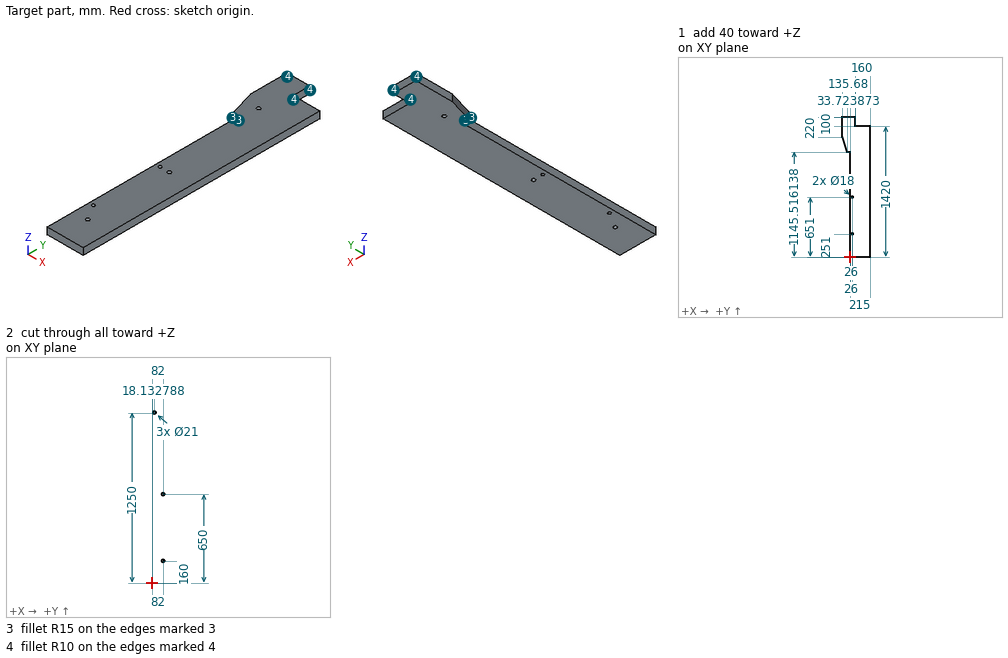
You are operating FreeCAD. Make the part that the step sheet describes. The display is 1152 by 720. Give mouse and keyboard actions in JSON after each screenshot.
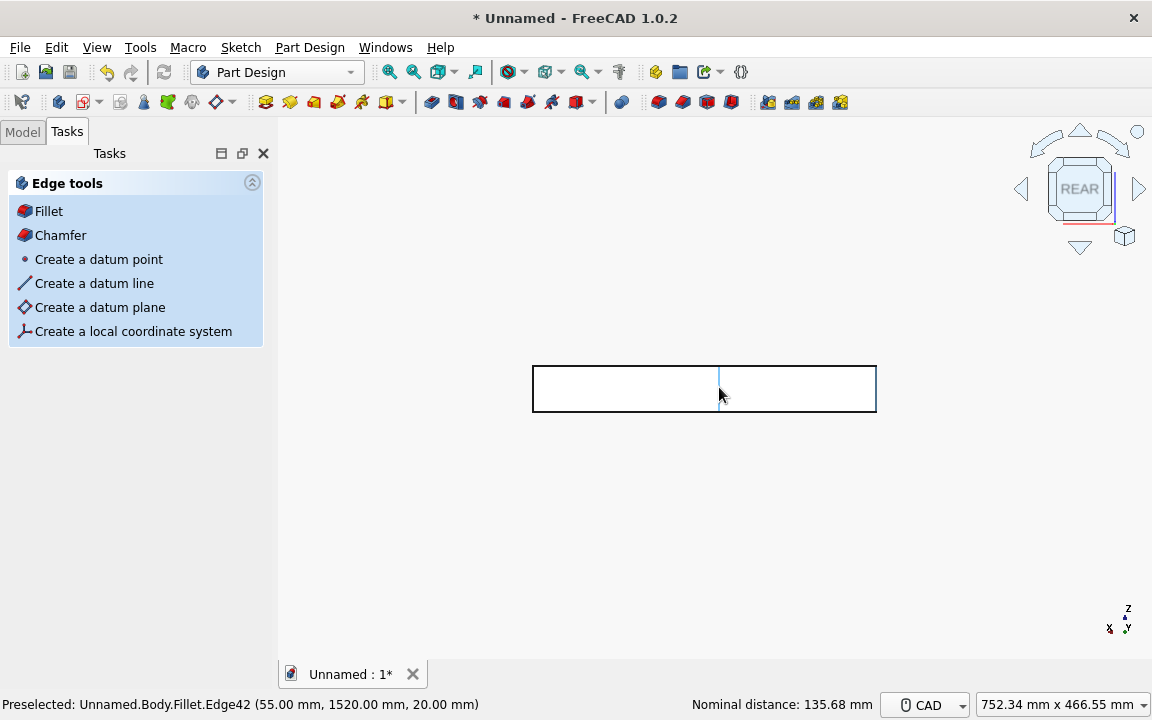
{"action": "key", "text": "v f"}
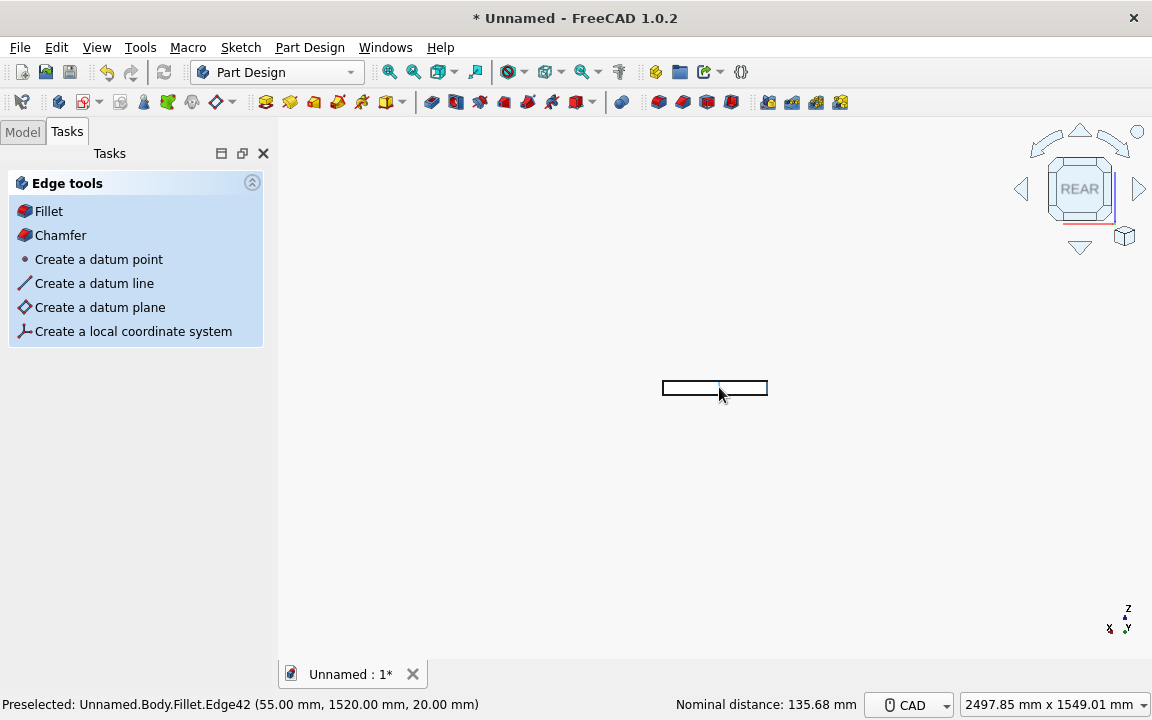
{"action": "key", "text": "6"}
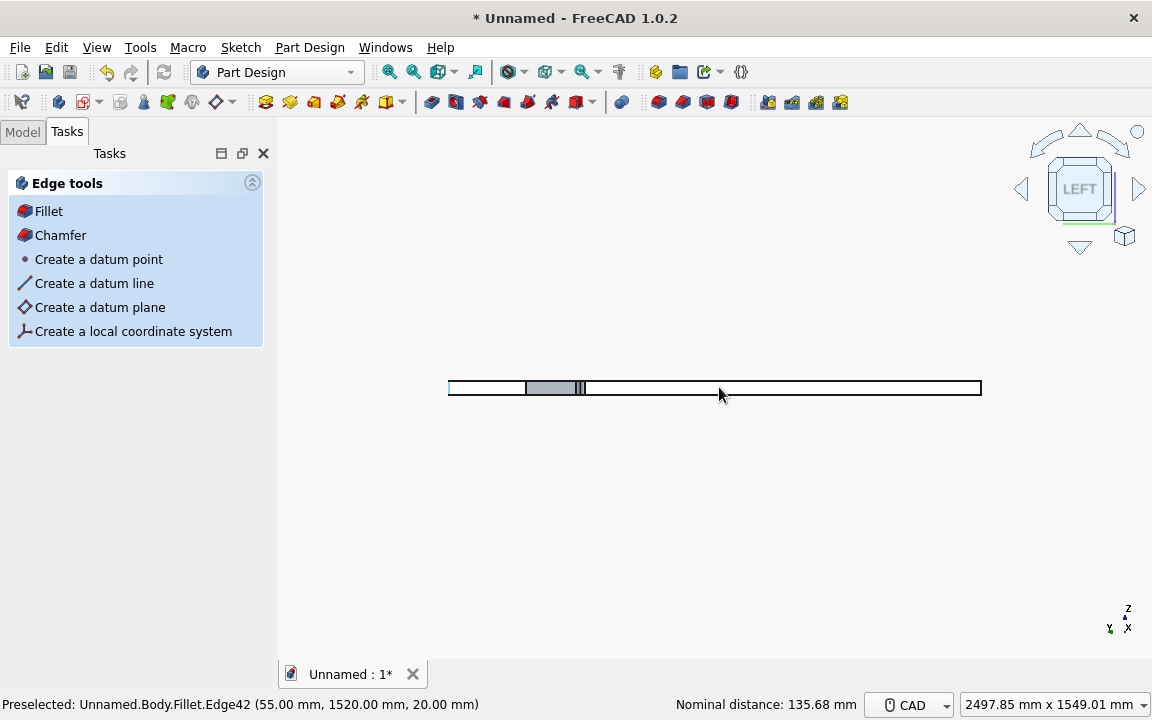
{"action": "scroll", "coordinate": [484, 387], "scroll_direction": "up", "scroll_amount": 6}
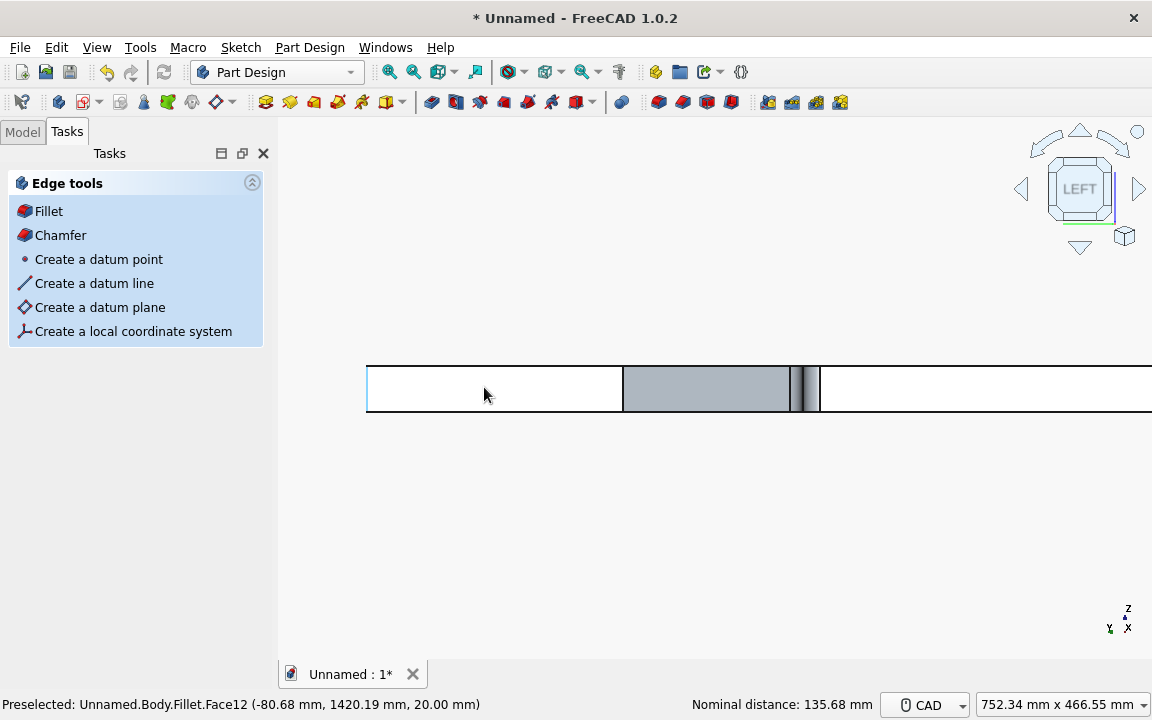
{"action": "key", "text": "v f"}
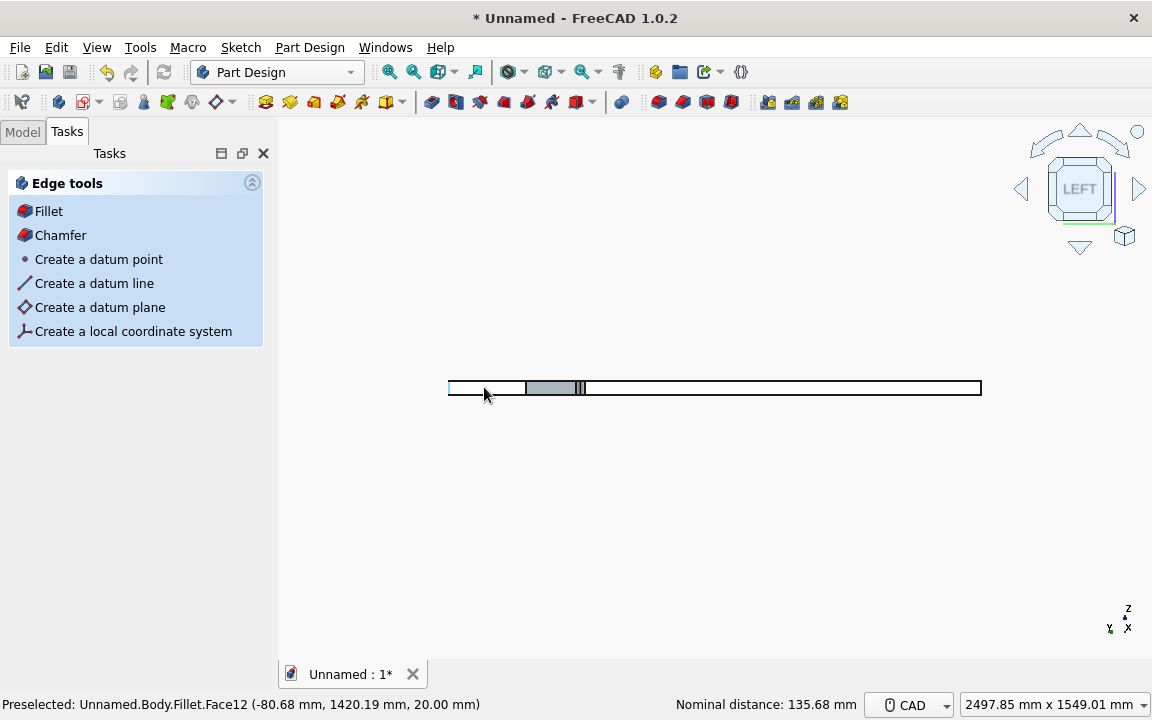
{"action": "key", "text": "v 3"}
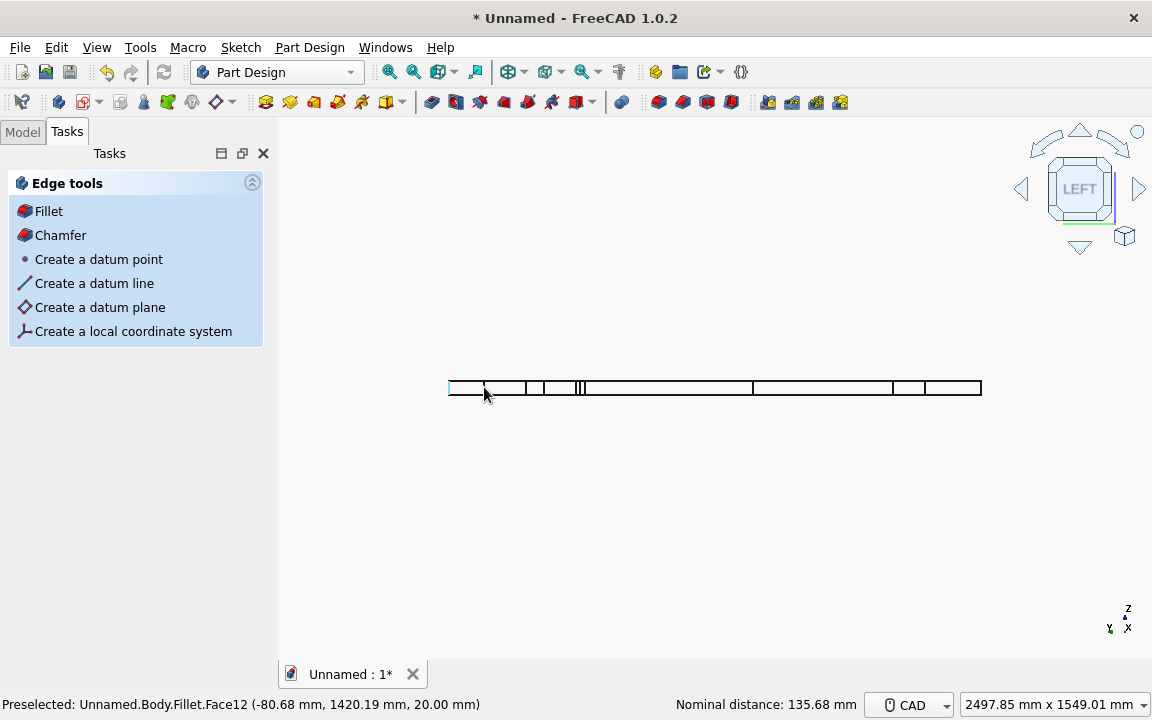
{"action": "key", "text": "0"}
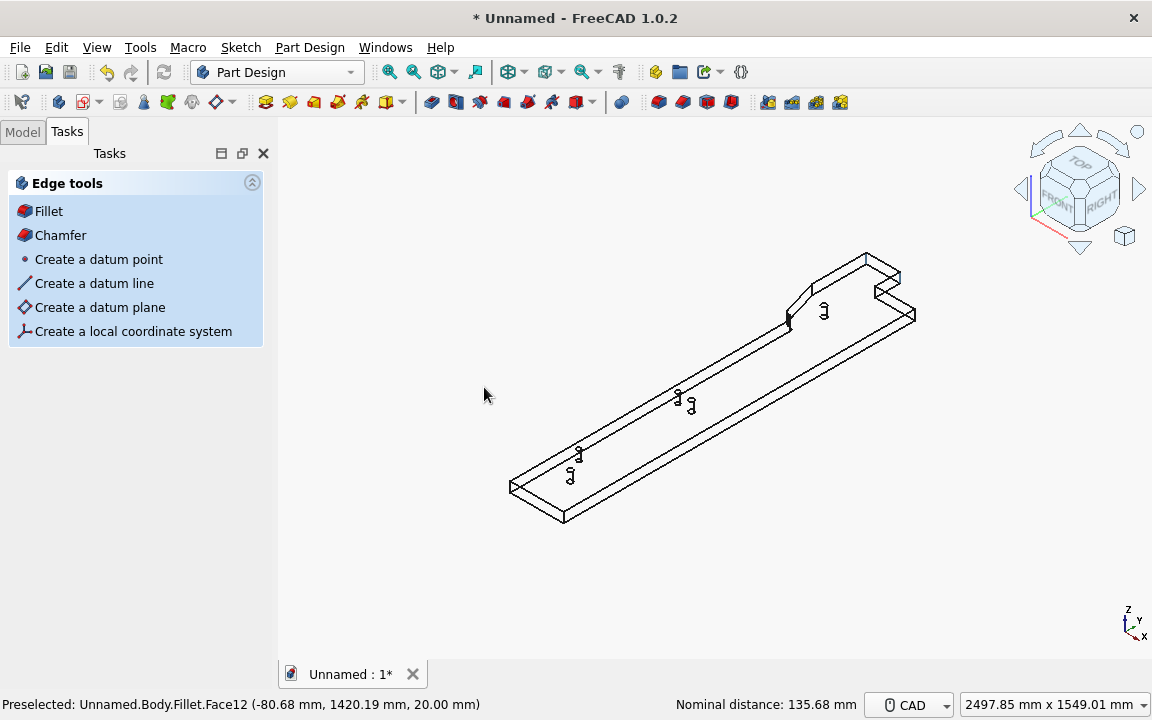
{"action": "left_click", "coordinate": [875, 293], "text": "ctrl"}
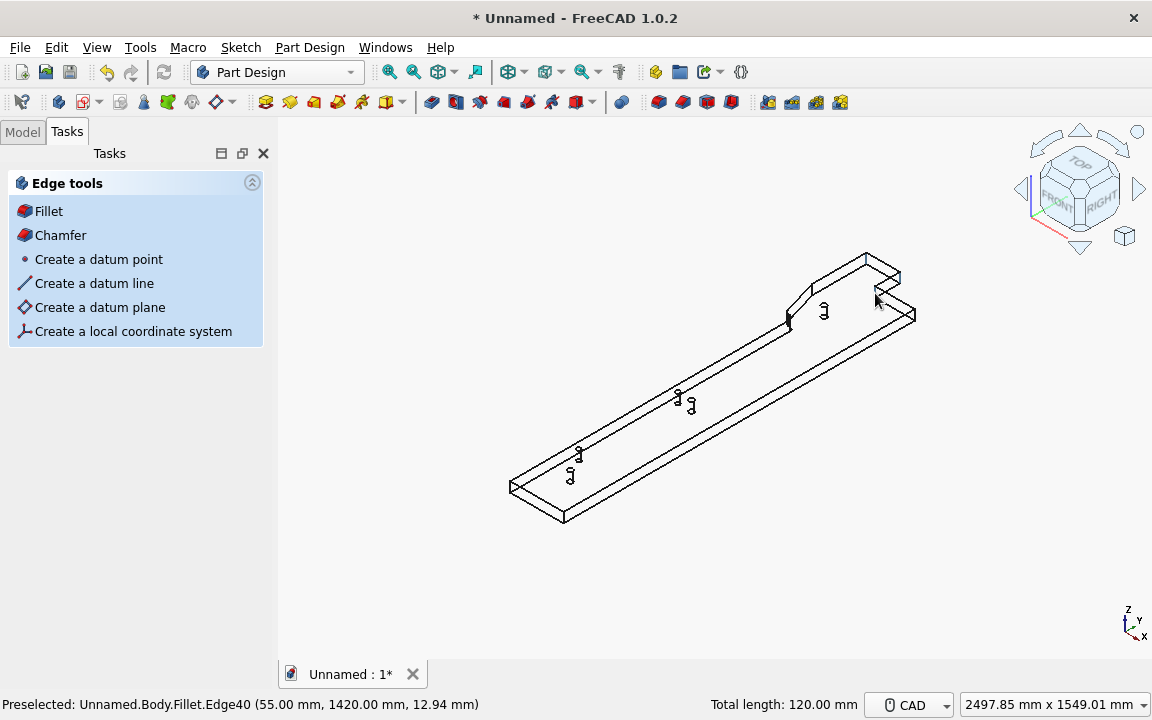
{"action": "key", "text": "v 1"}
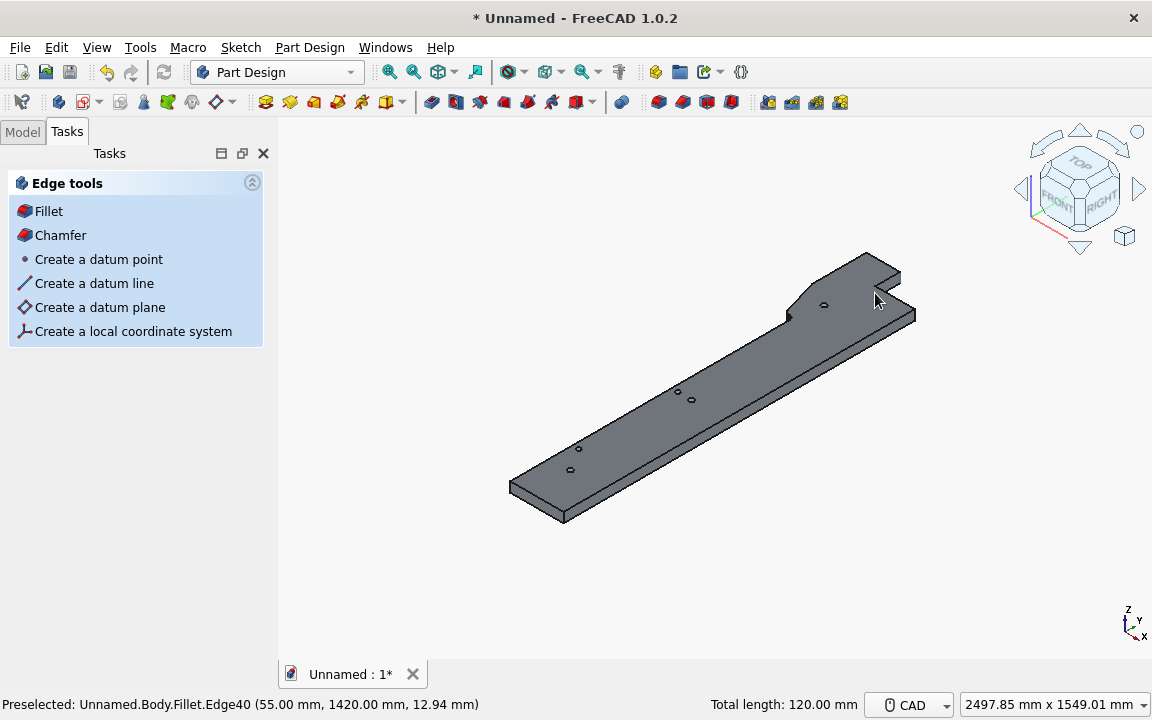
{"action": "left_click", "coordinate": [660, 102]}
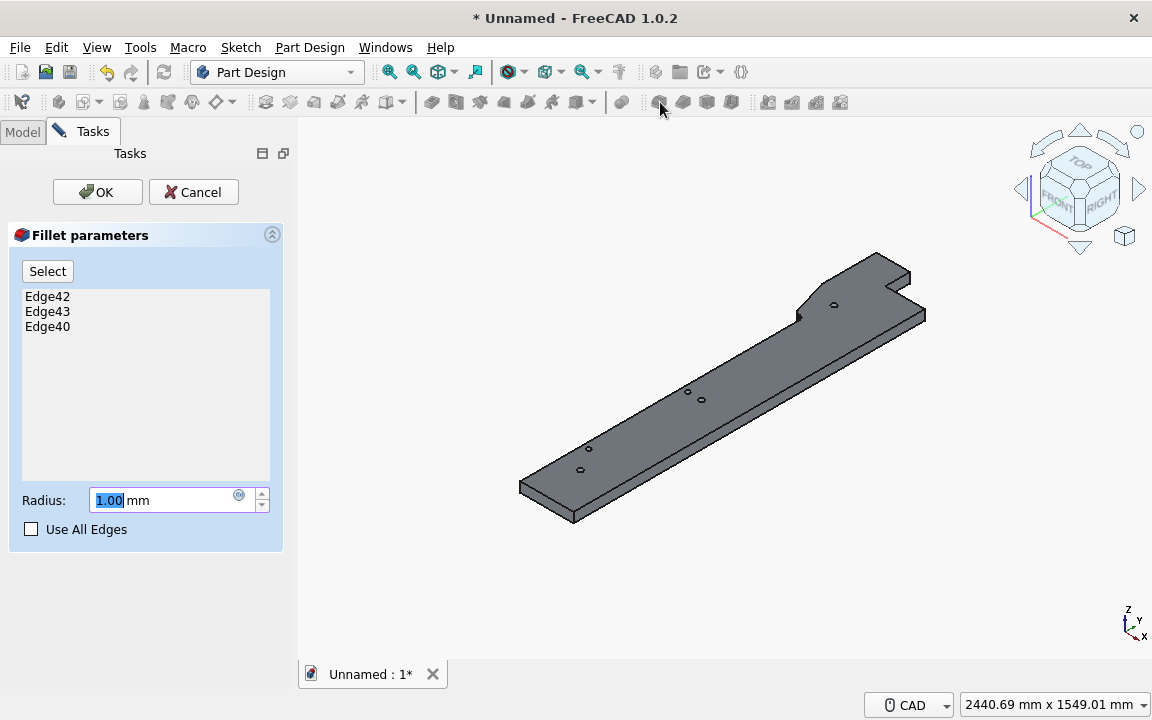
{"action": "type", "text": "10"}
{"action": "key", "text": "Tab"}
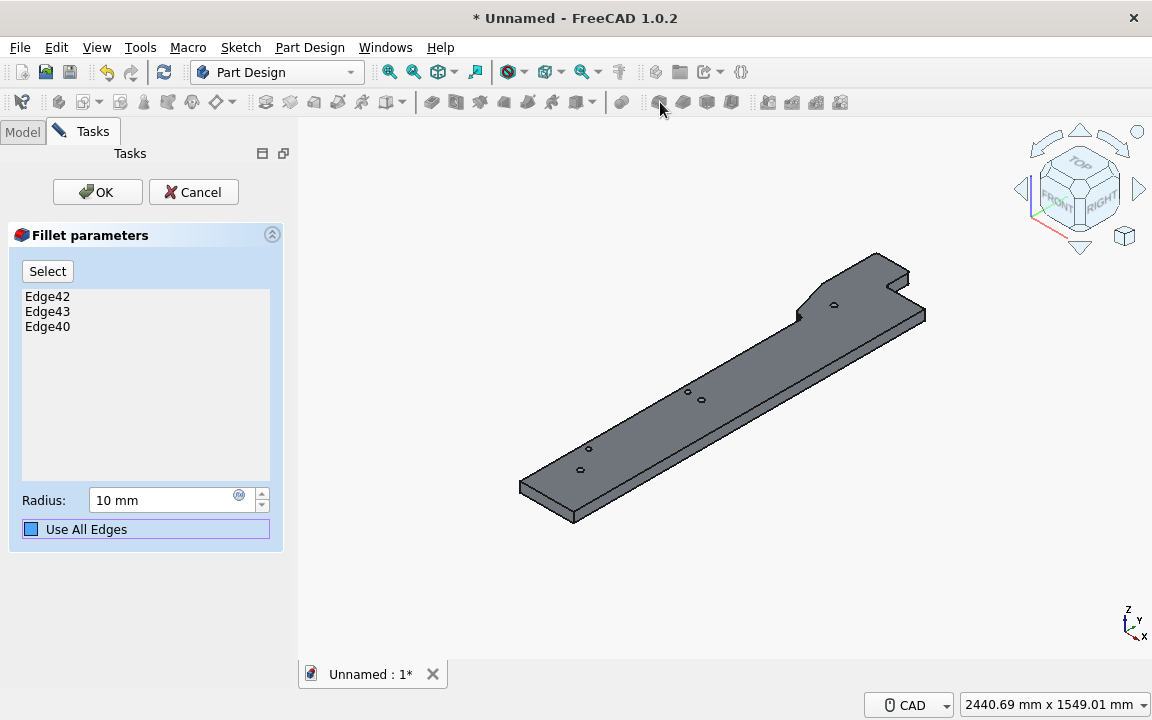
{"action": "left_click", "coordinate": [98, 192]}